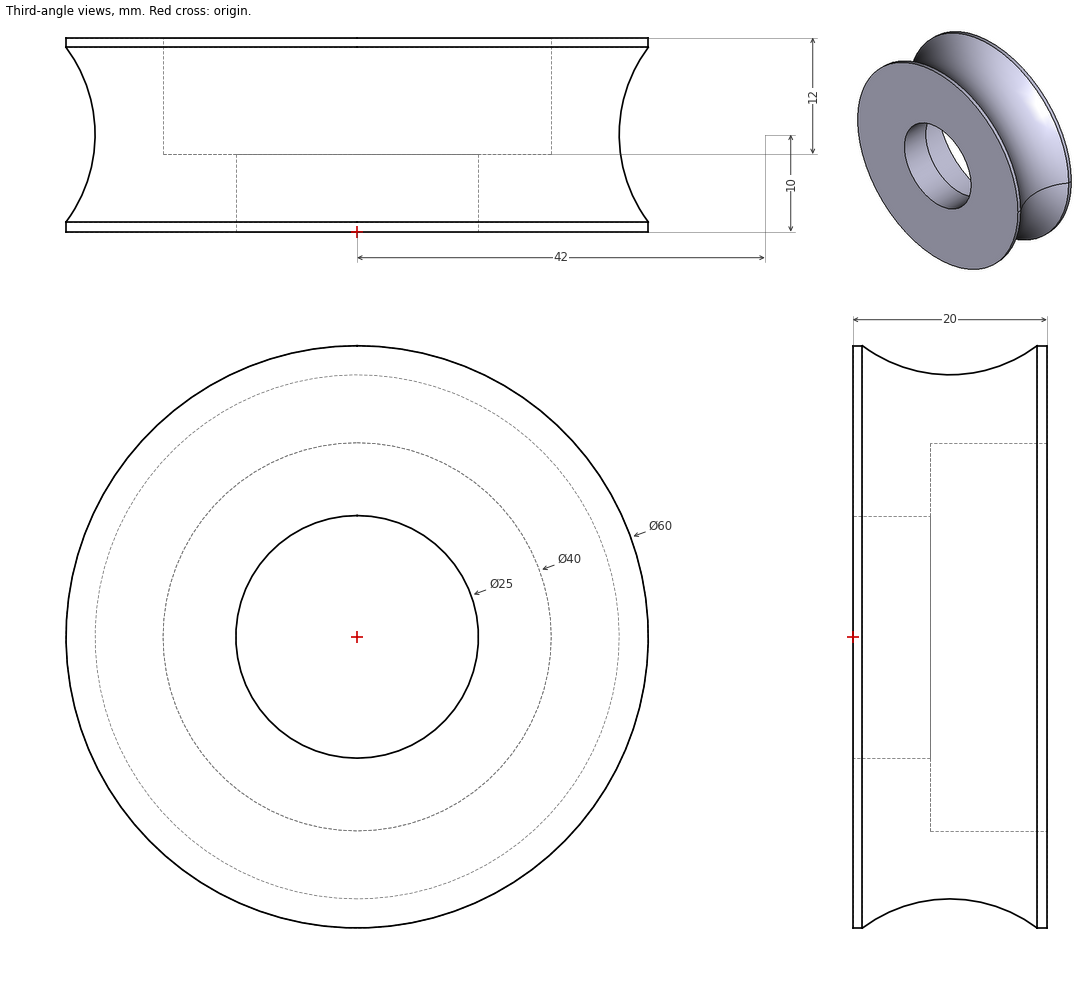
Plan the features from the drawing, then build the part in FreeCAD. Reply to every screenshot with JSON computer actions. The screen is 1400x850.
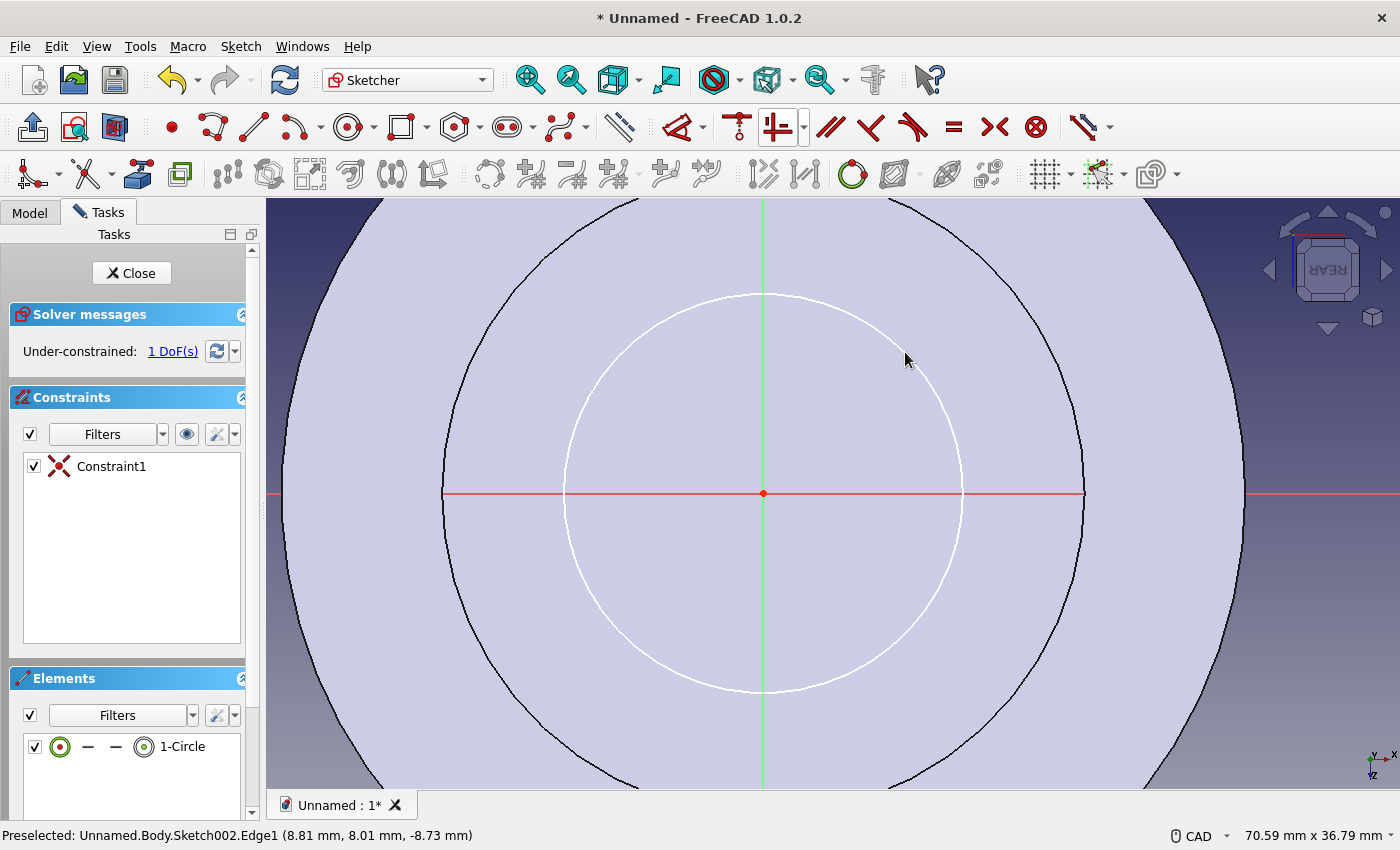
{"action": "left_click", "coordinate": [676, 128]}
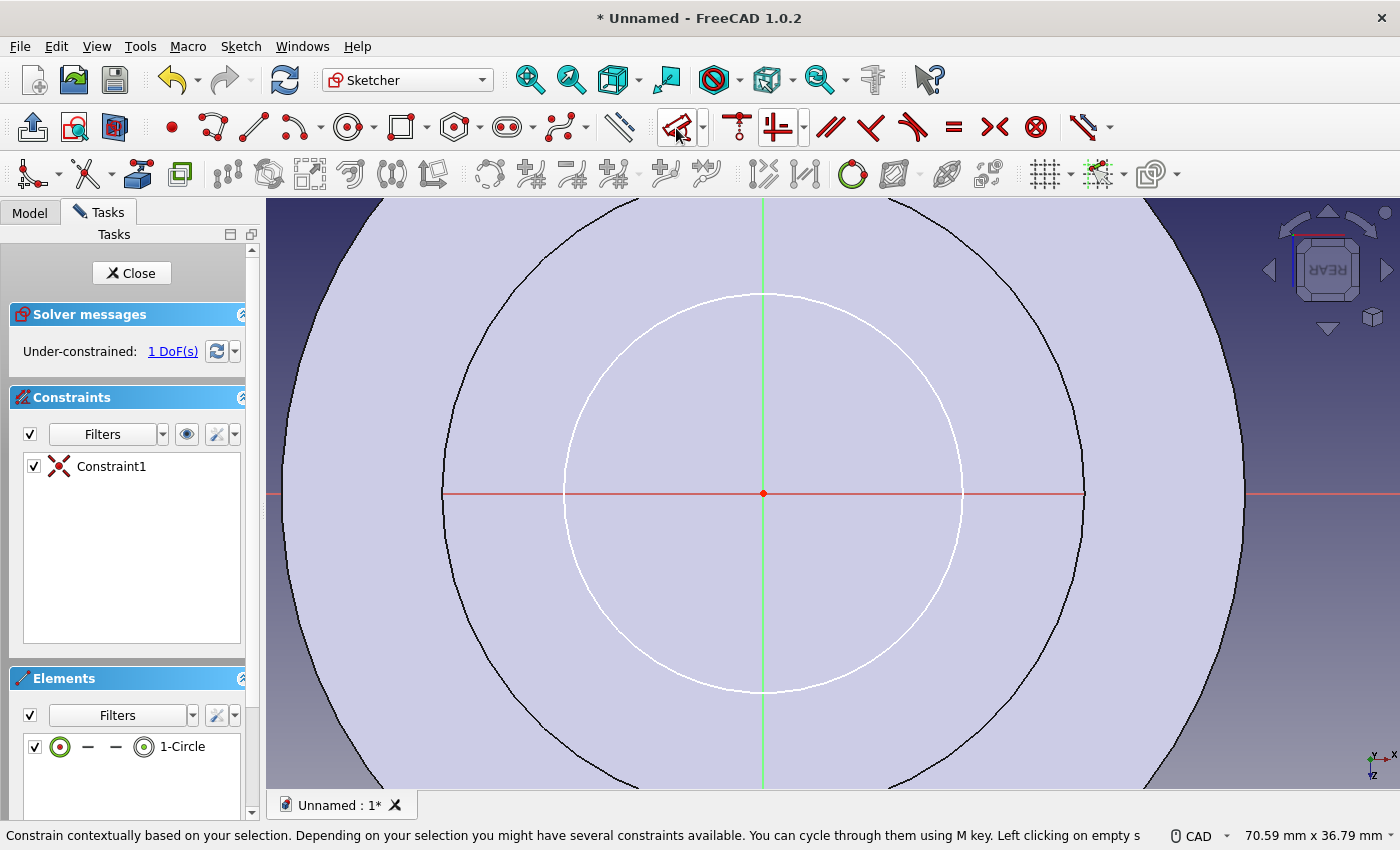
{"action": "left_click", "coordinate": [904, 352]}
{"action": "left_click", "coordinate": [927, 329]}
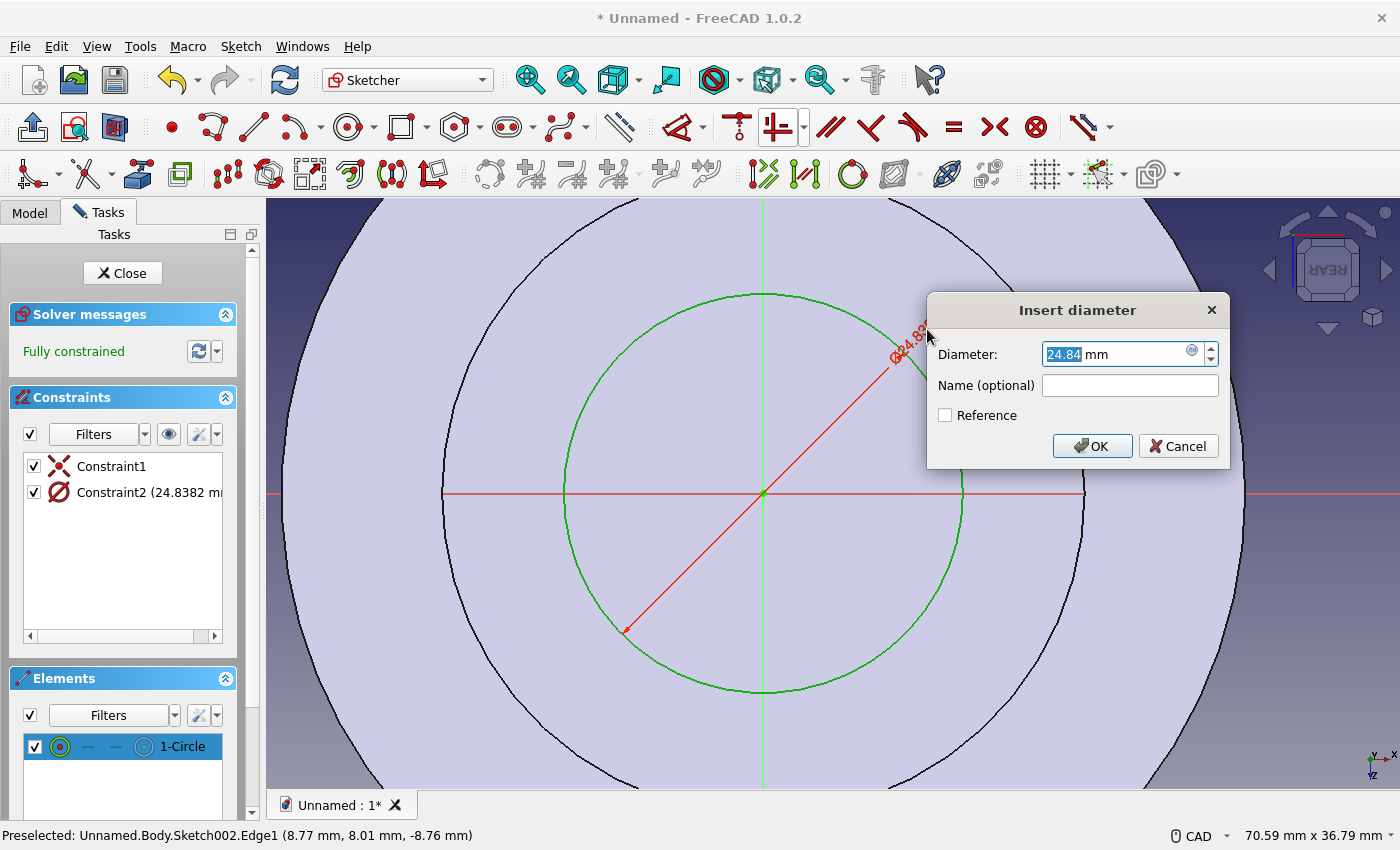
{"action": "type", "text": "25"}
{"action": "key", "text": "Return"}
{"action": "key", "text": "Escape"}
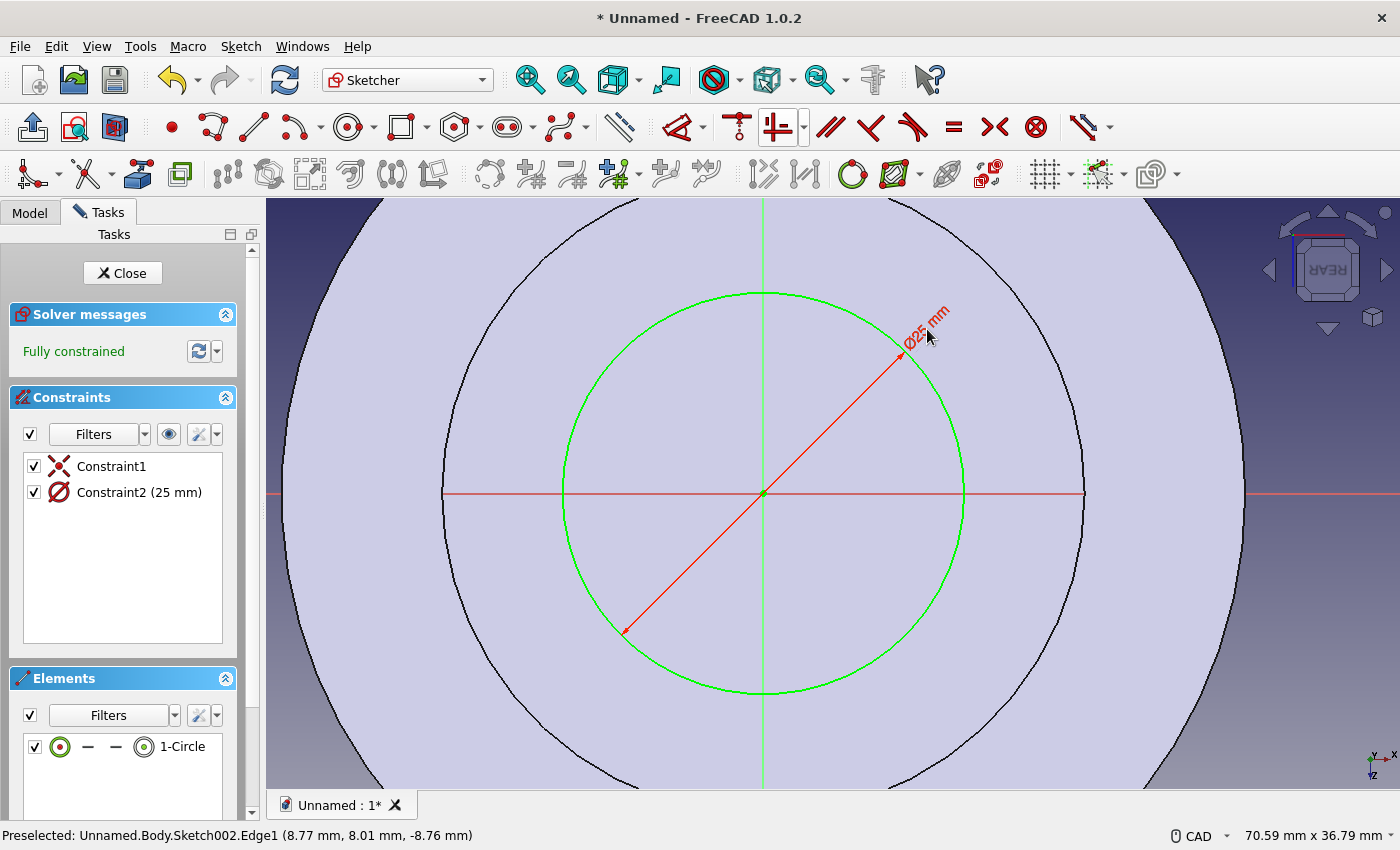
{"action": "left_click", "coordinate": [123, 273]}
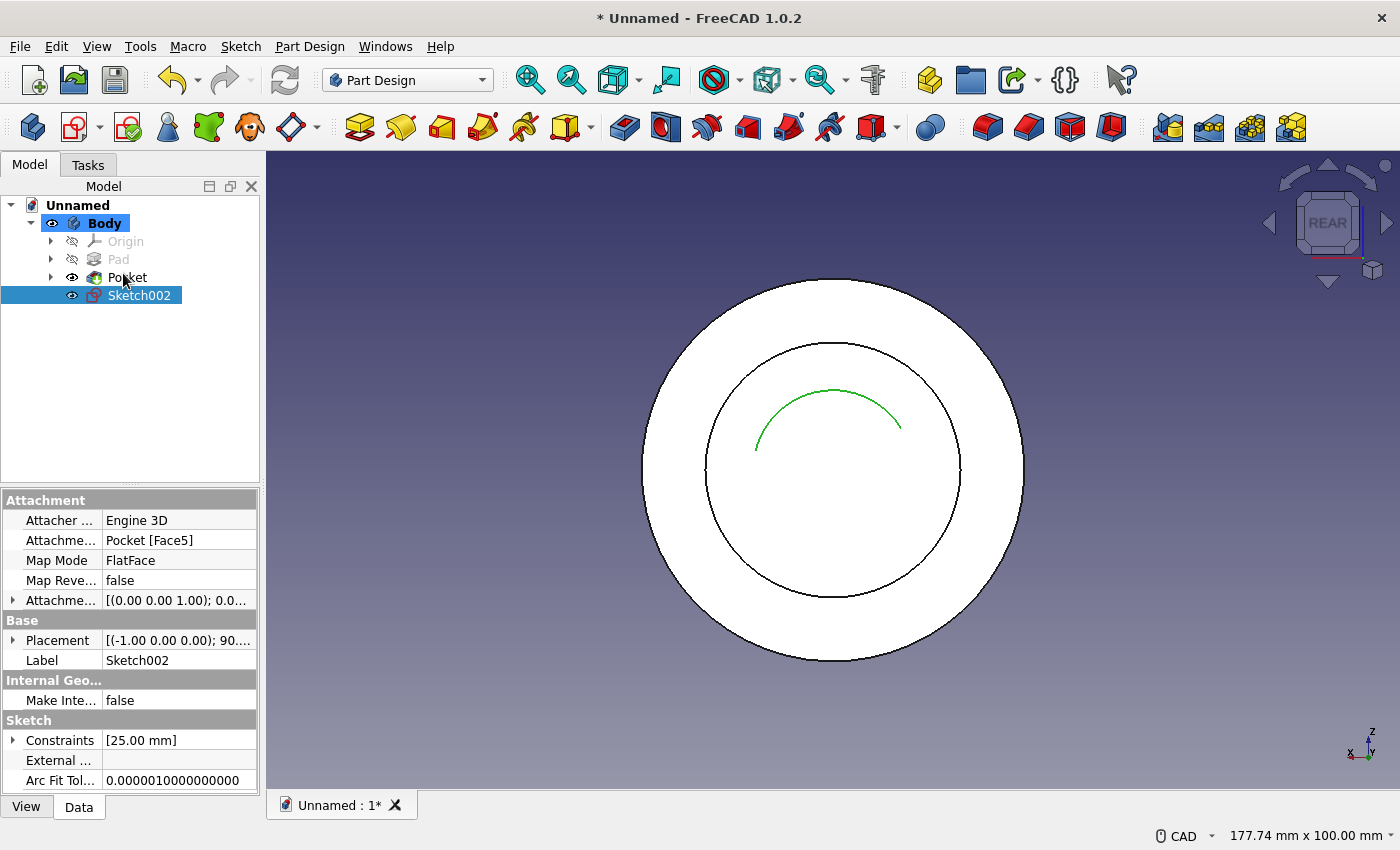
{"action": "left_click", "coordinate": [625, 128]}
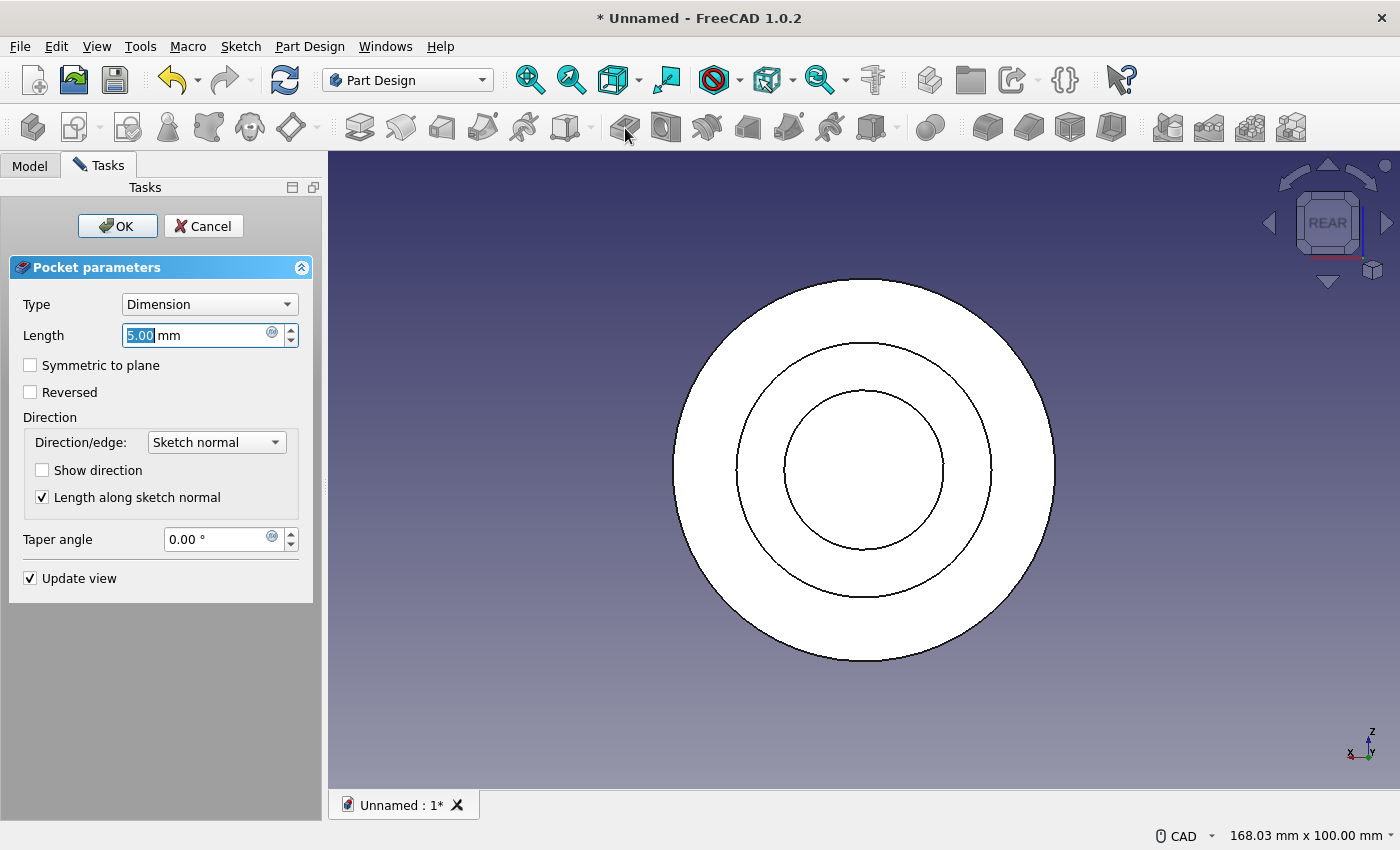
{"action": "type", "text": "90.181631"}
{"action": "key", "text": "Tab"}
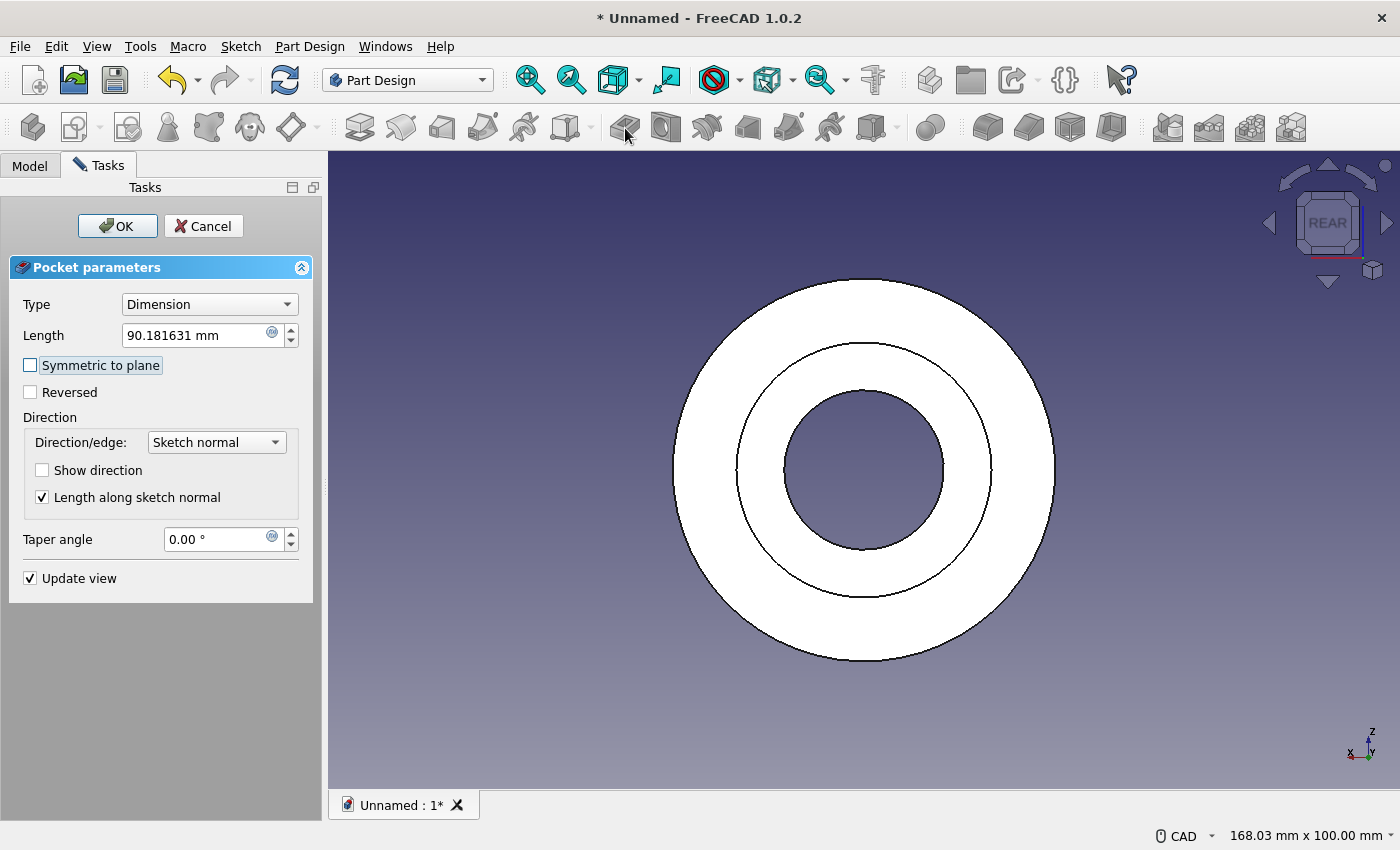
{"action": "left_click", "coordinate": [31, 365]}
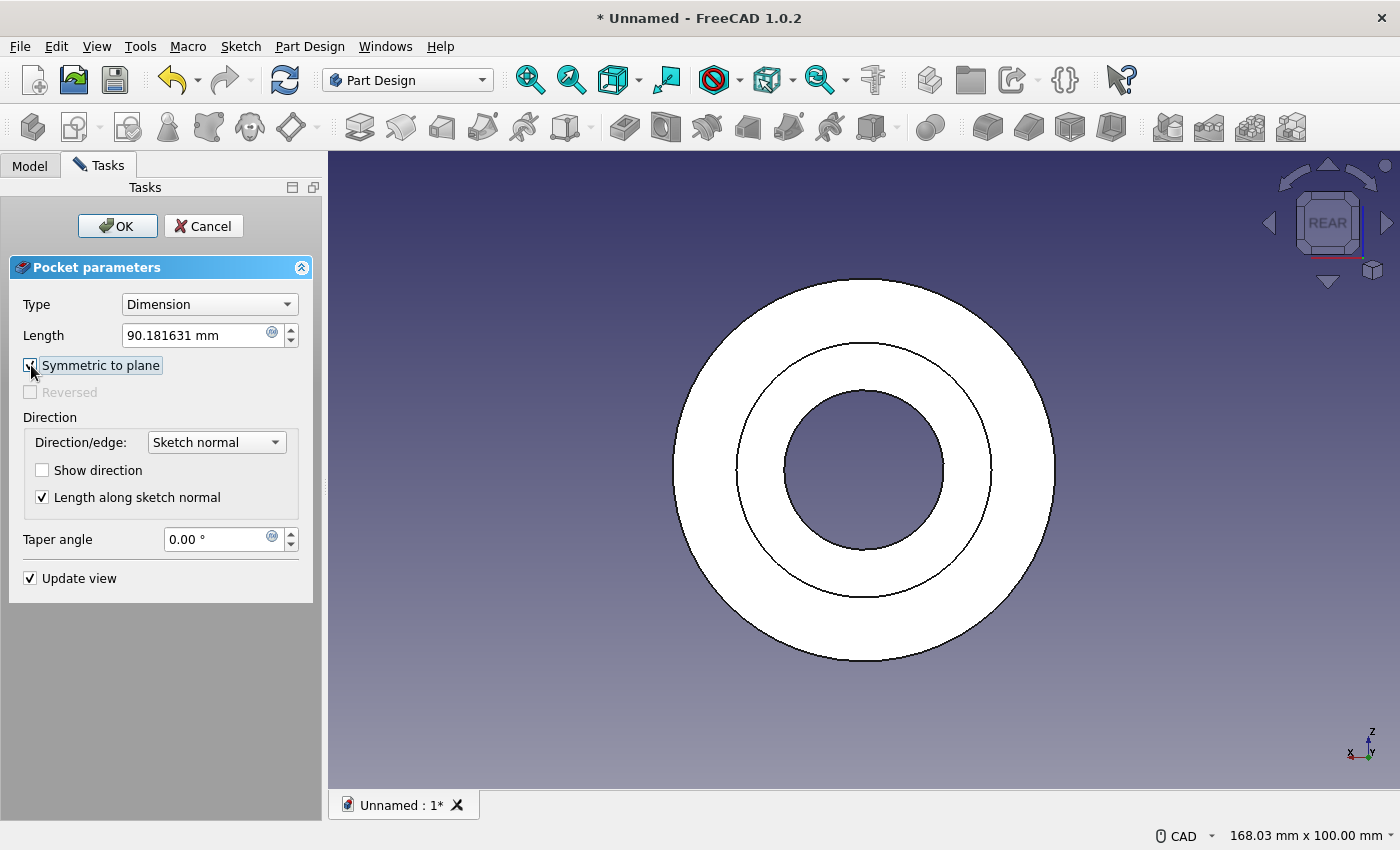
{"action": "left_click", "coordinate": [118, 226]}